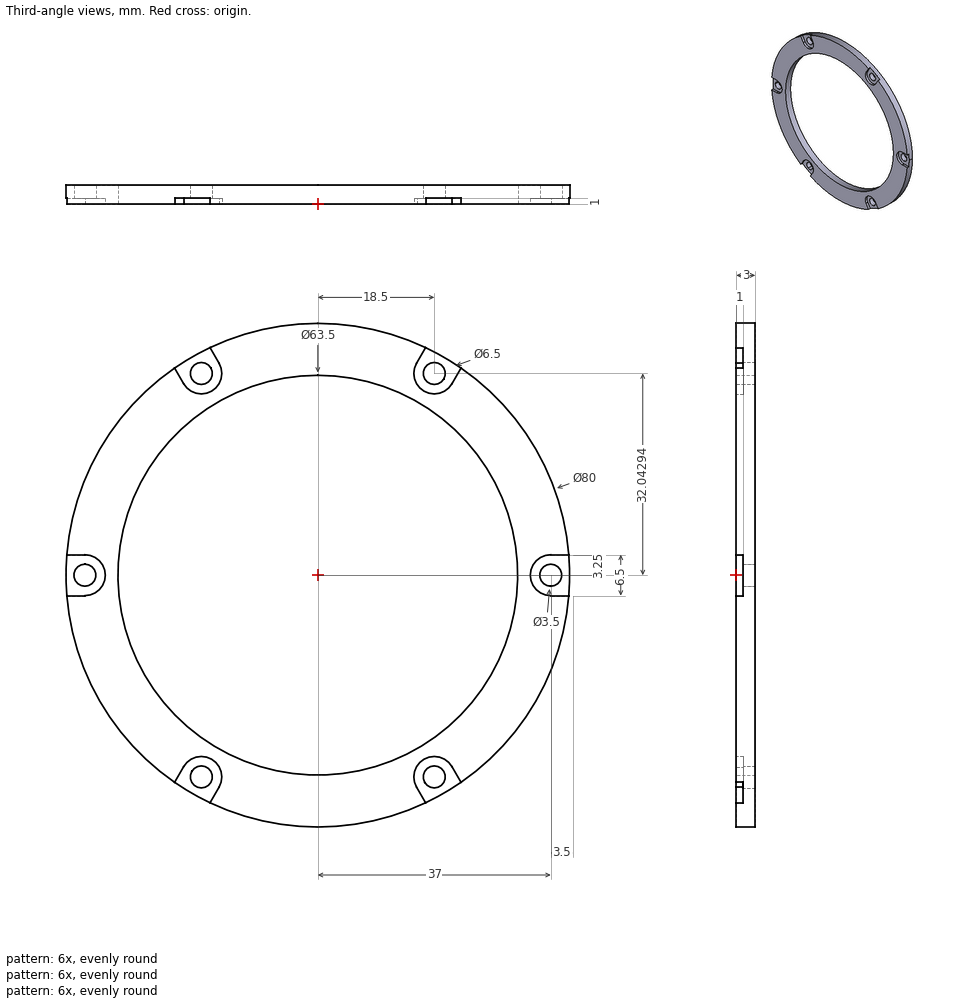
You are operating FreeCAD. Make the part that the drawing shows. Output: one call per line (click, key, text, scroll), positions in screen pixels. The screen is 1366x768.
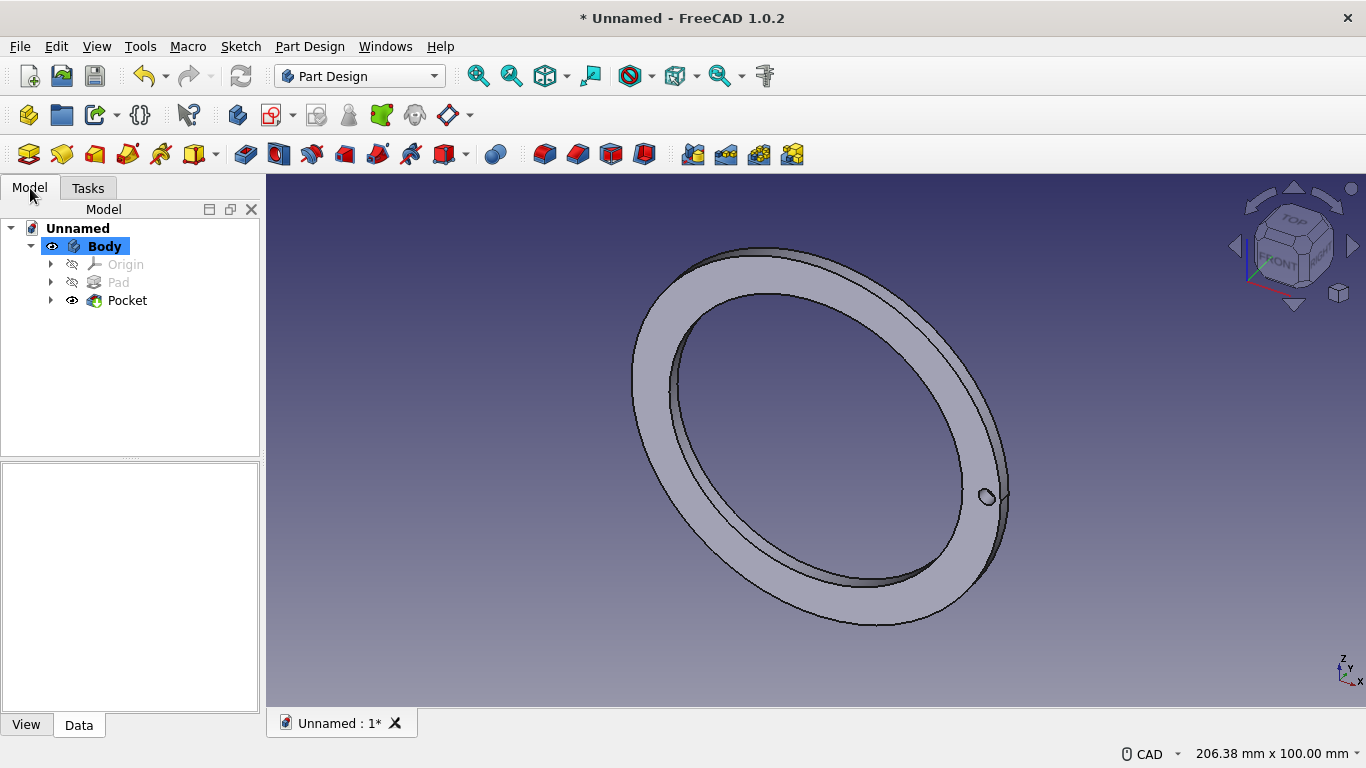
click(117, 300)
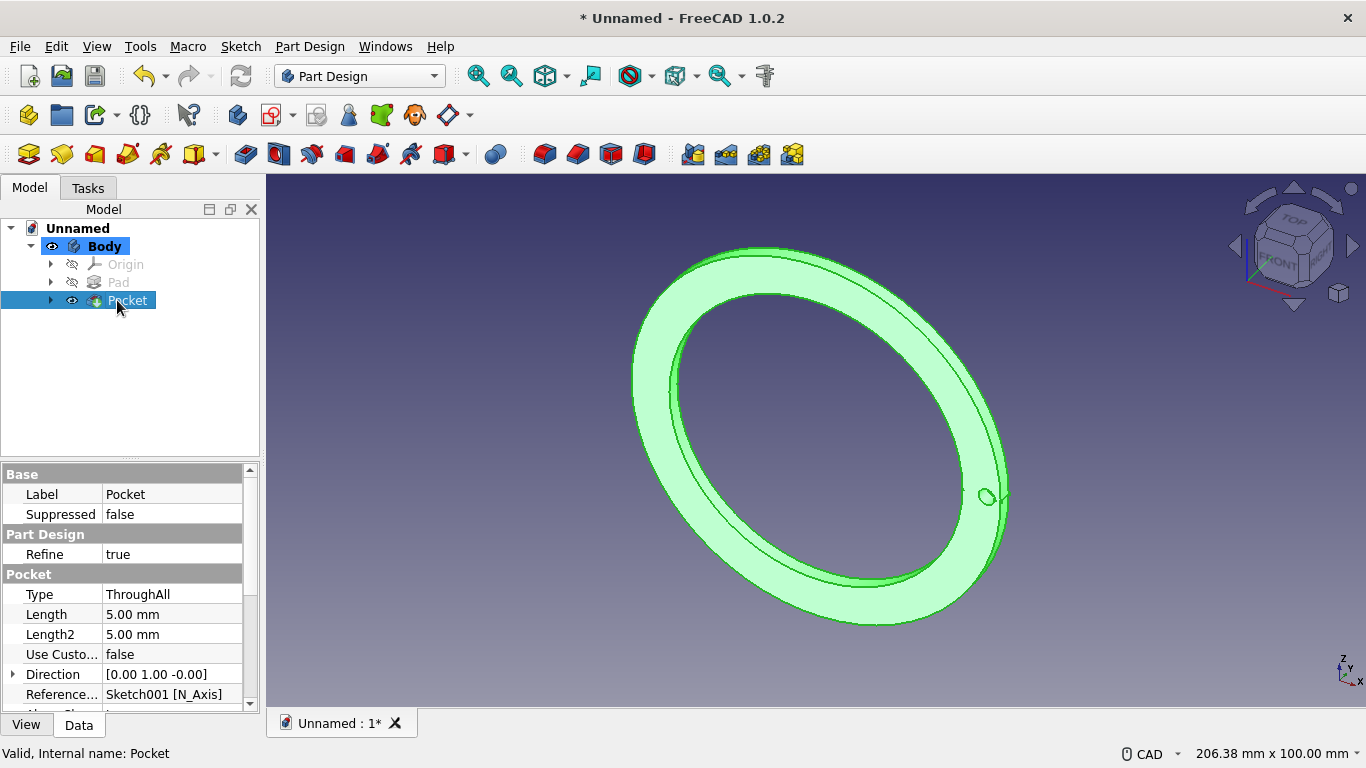
click(759, 154)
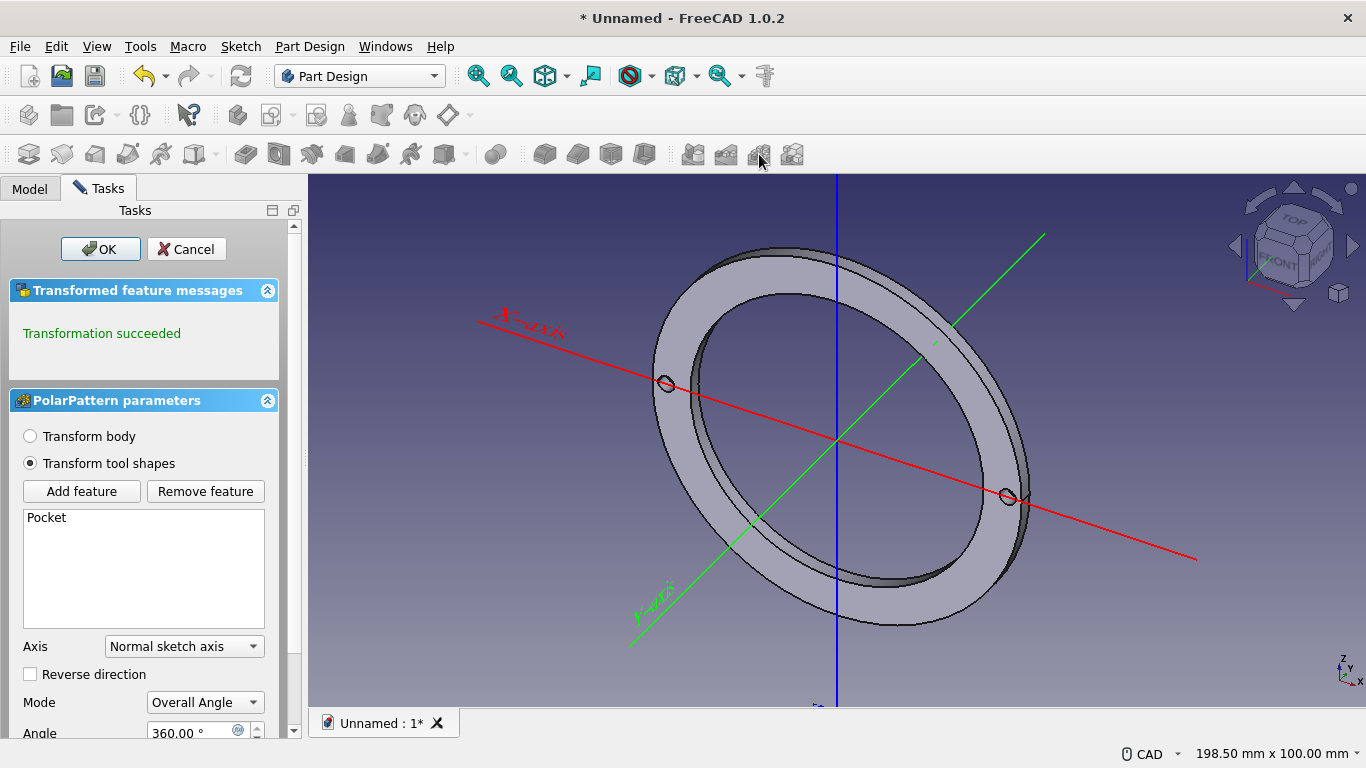
click(185, 646)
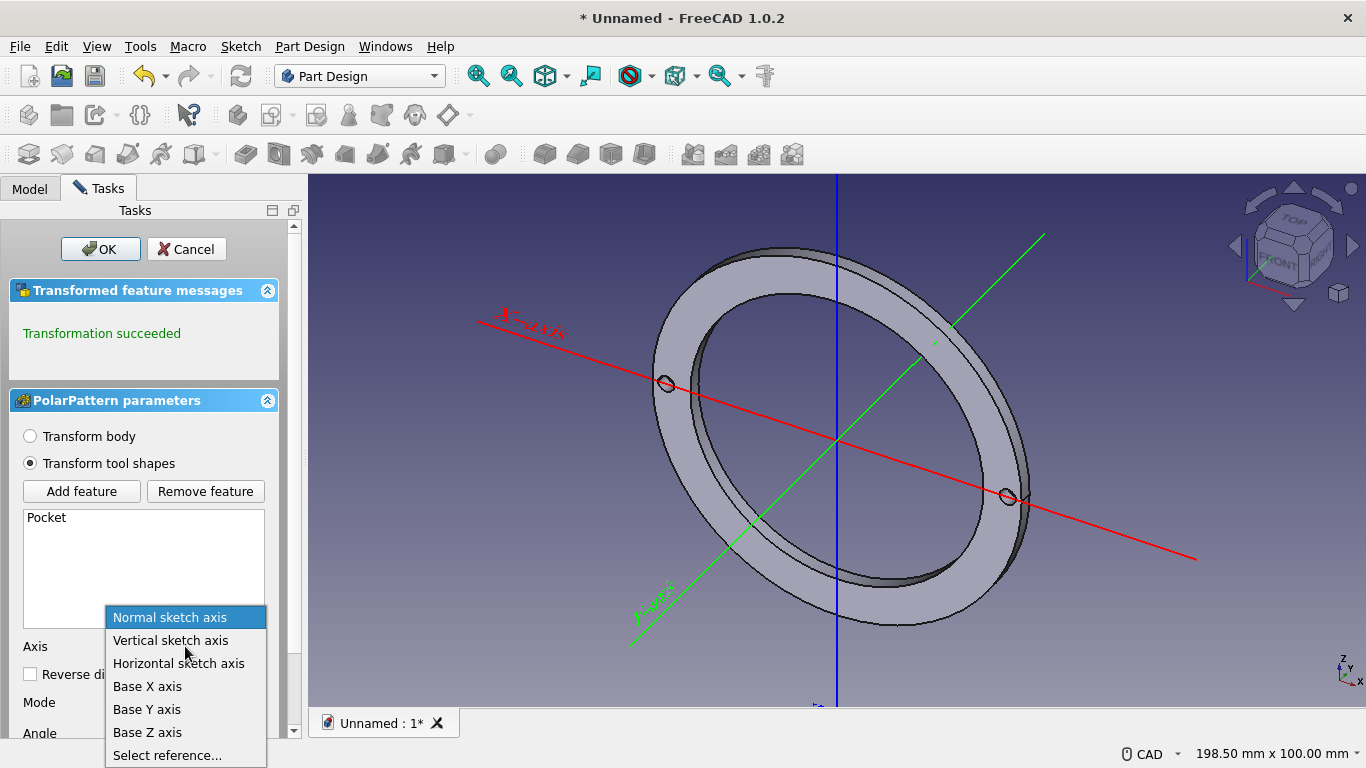
click(184, 710)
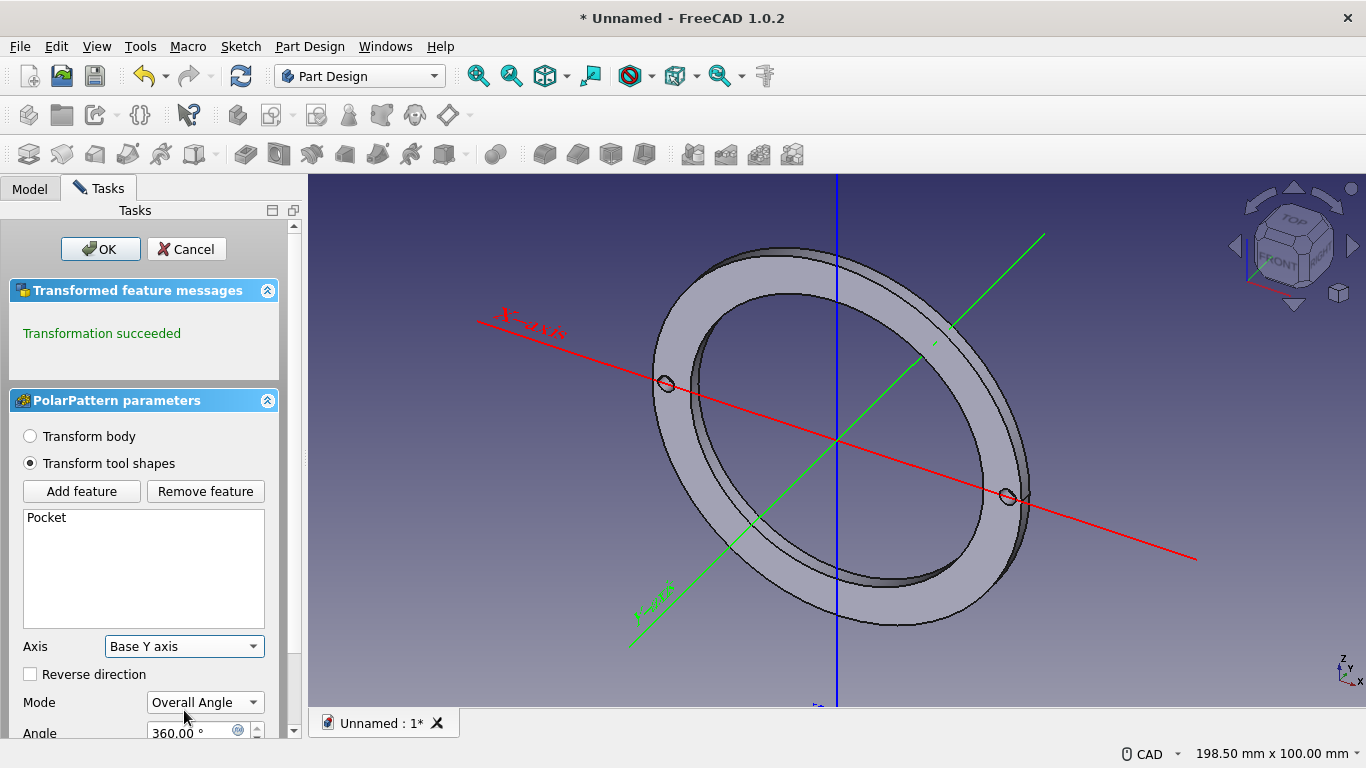
scroll(294, 479, down, 2)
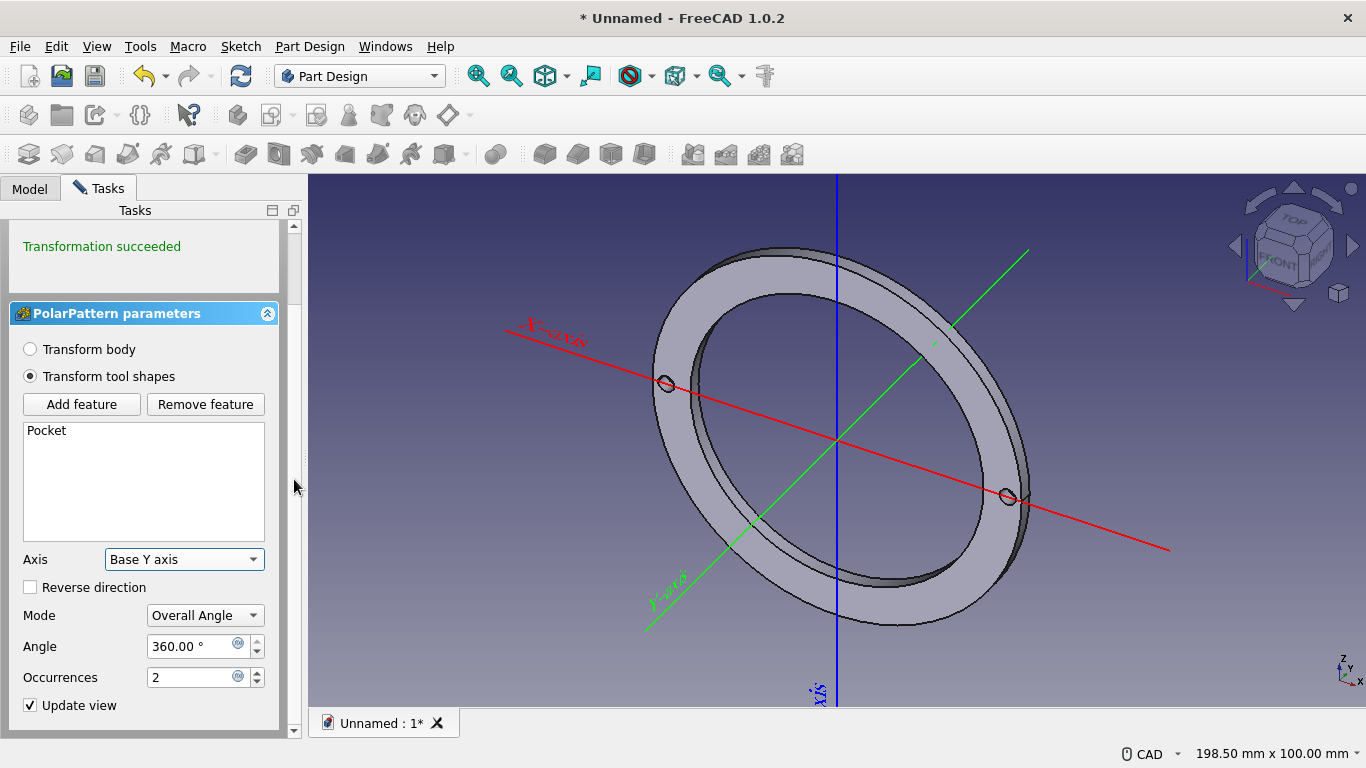
triple_click(199, 678)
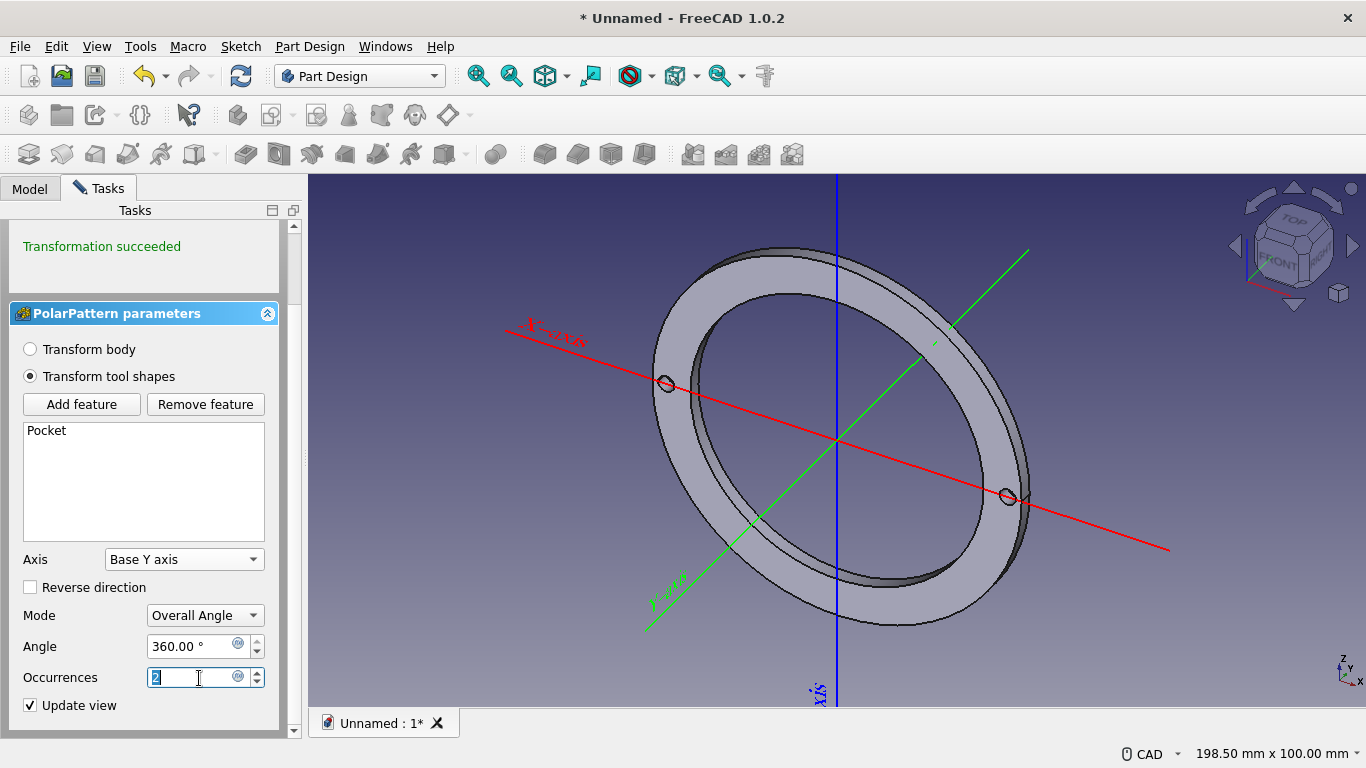
text(6)
key(Tab)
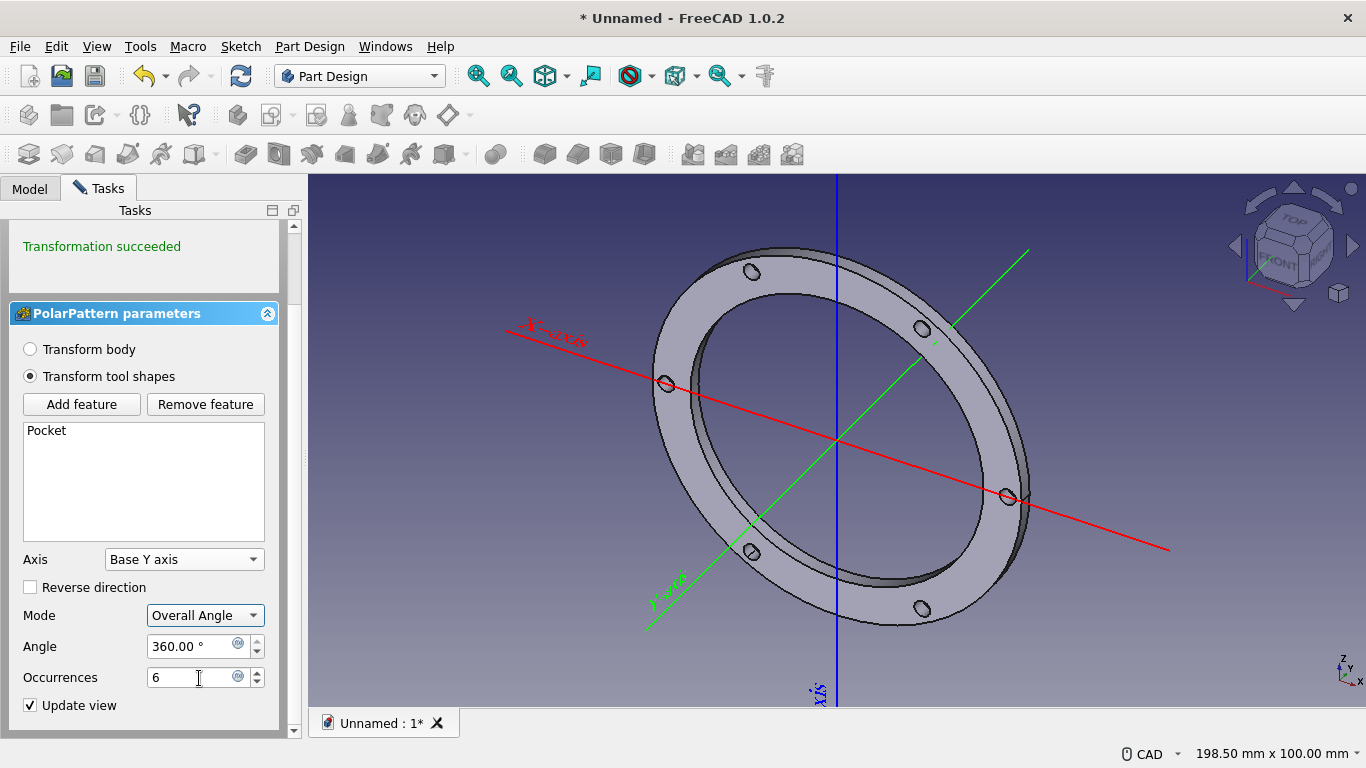
scroll(294, 479, up, 3)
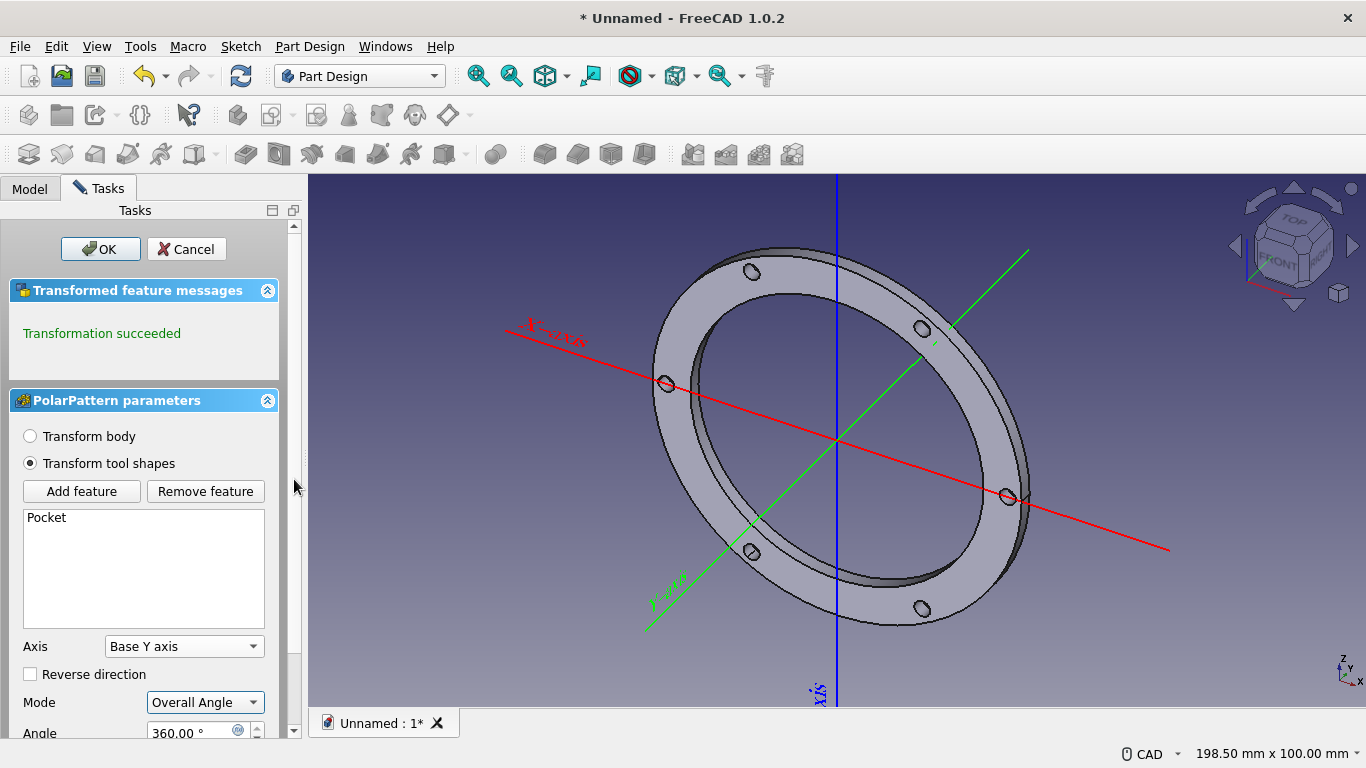
click(101, 249)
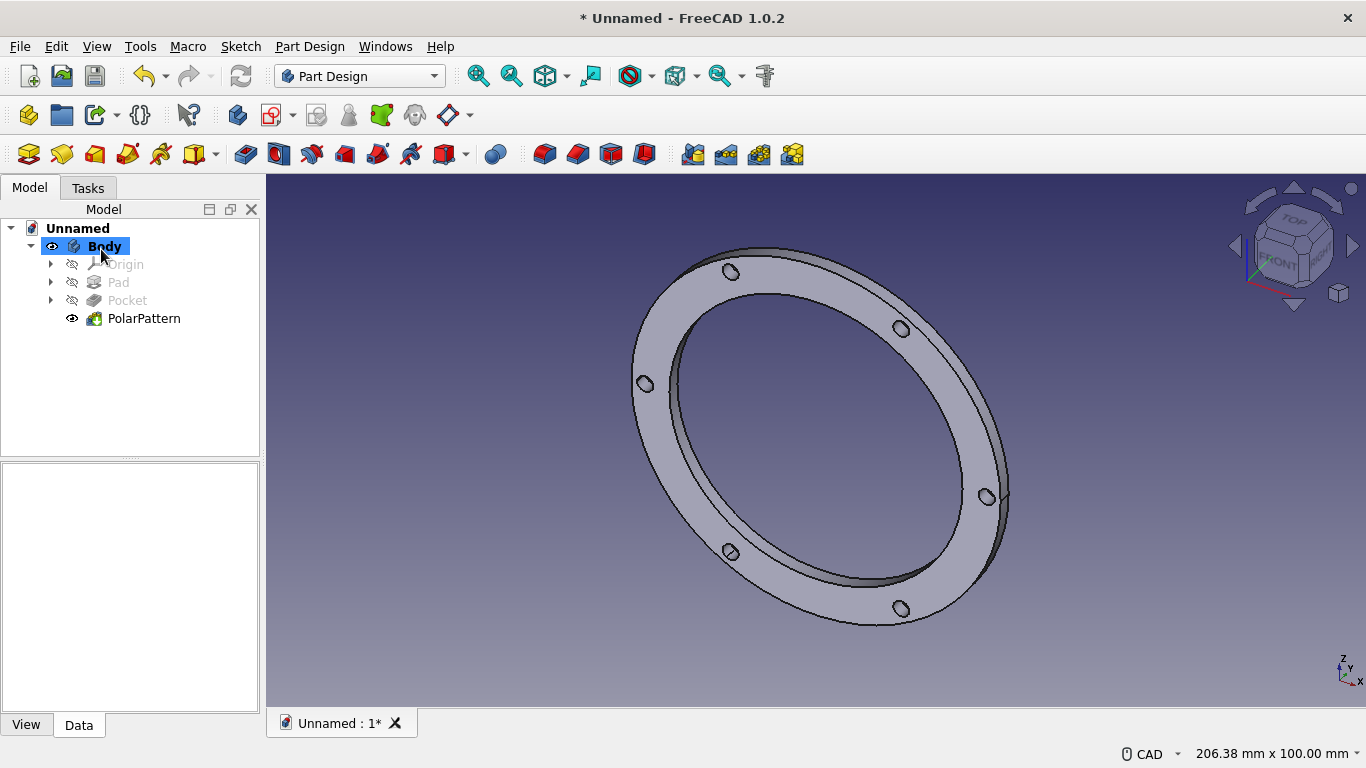
click(763, 572)